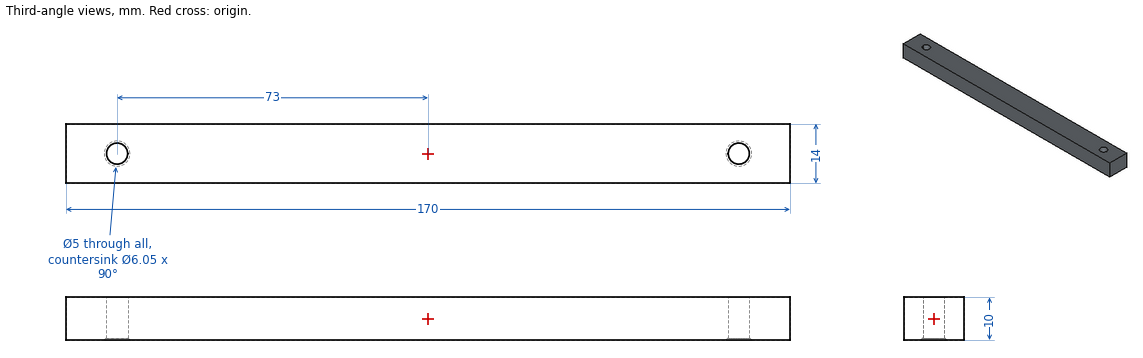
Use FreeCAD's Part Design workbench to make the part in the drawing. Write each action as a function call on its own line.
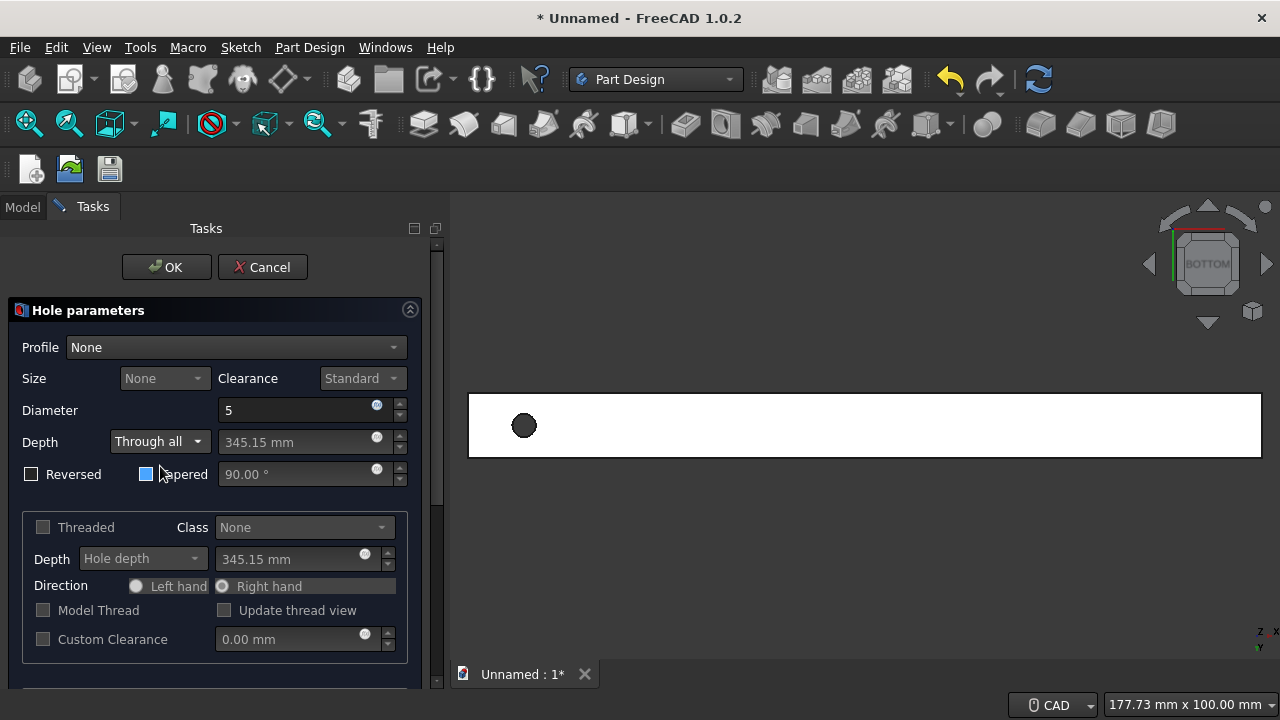
scroll(437, 463, down, 2)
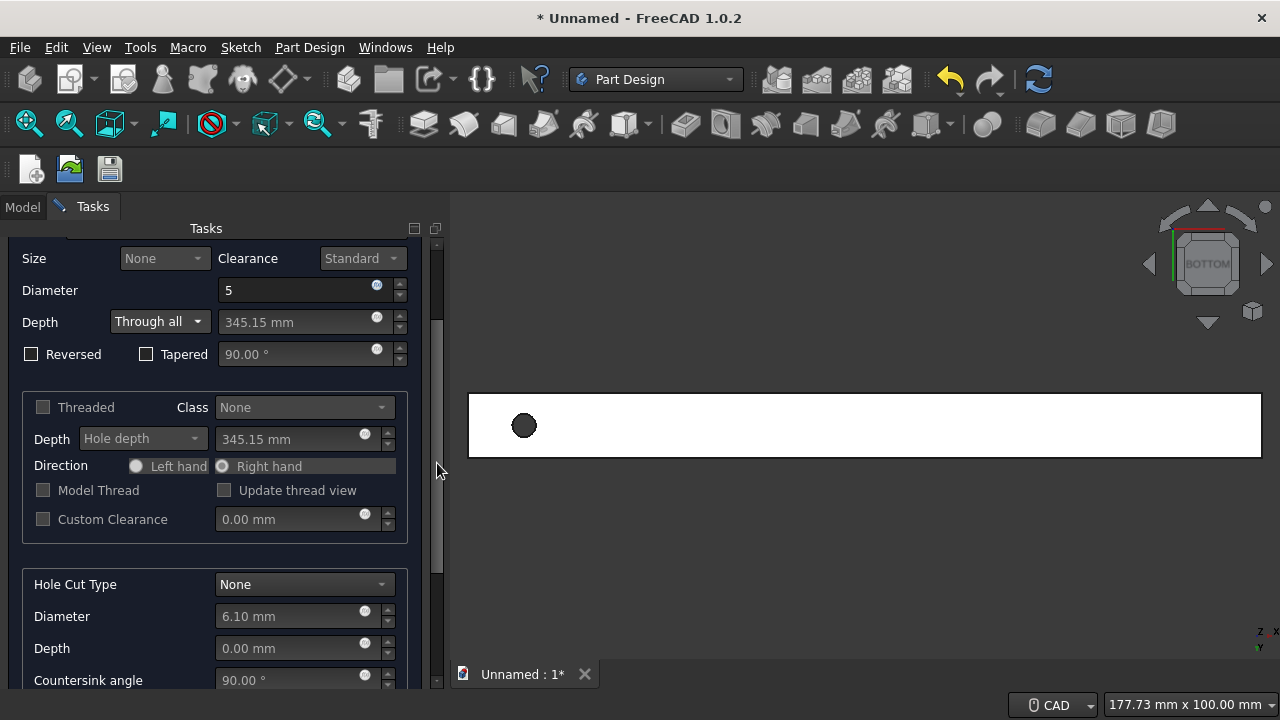
click(306, 584)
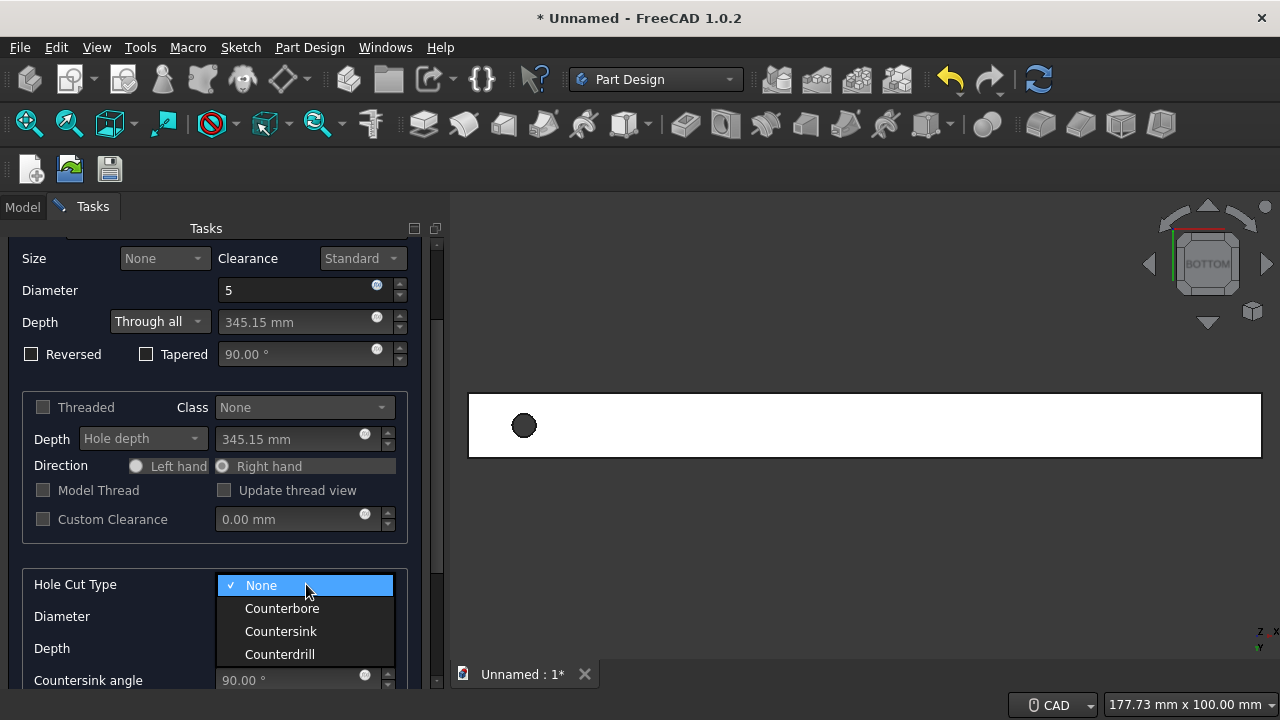
click(304, 632)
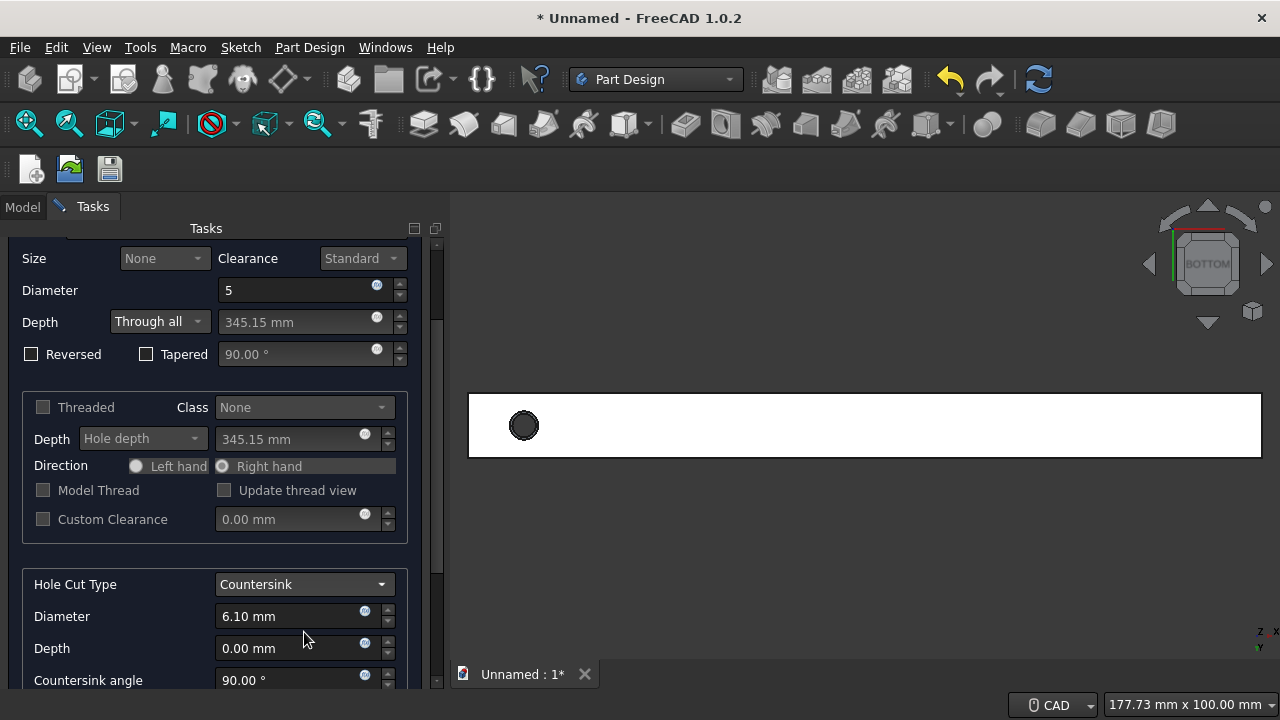
triple_click(298, 616)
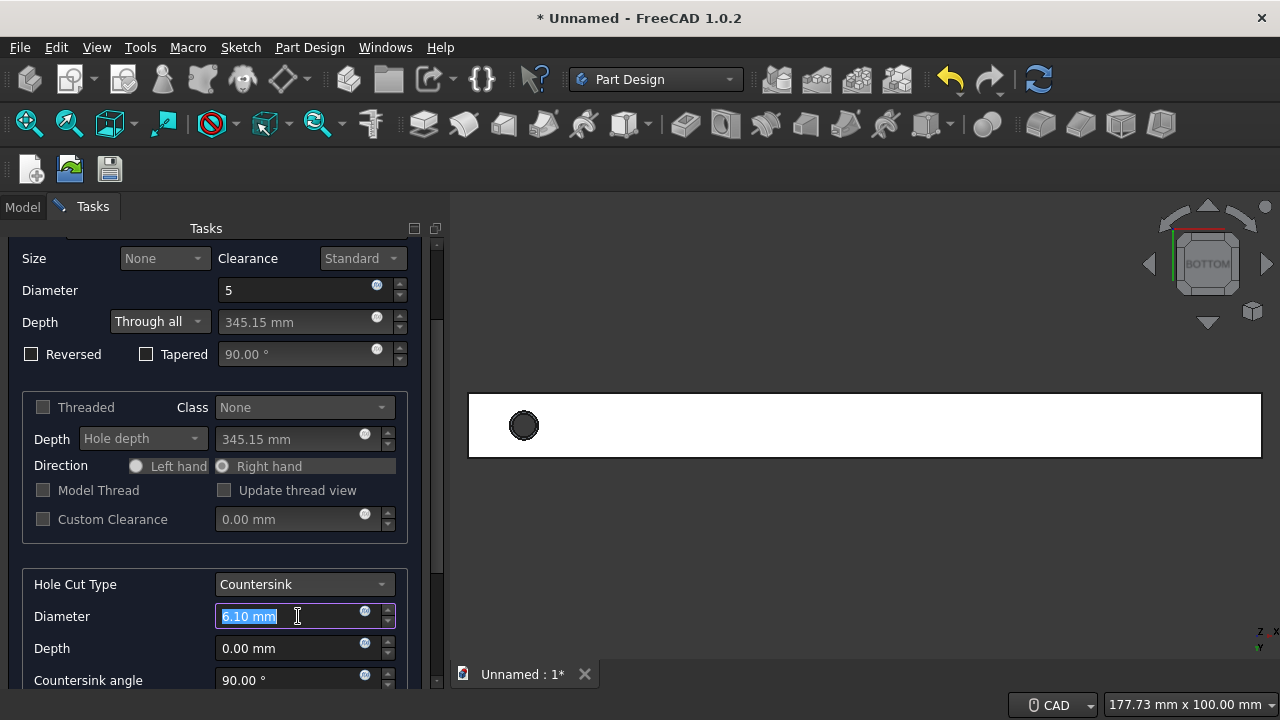
text(6.05)
key(Tab)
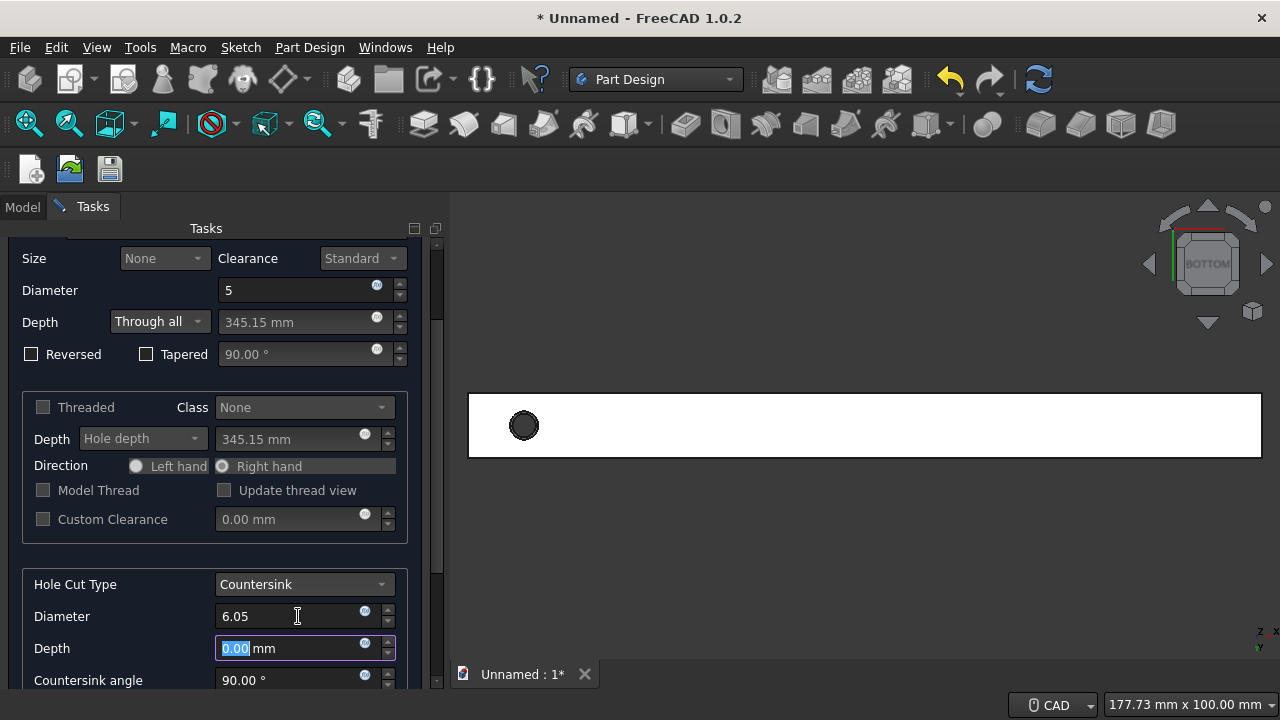
scroll(437, 463, up, 3)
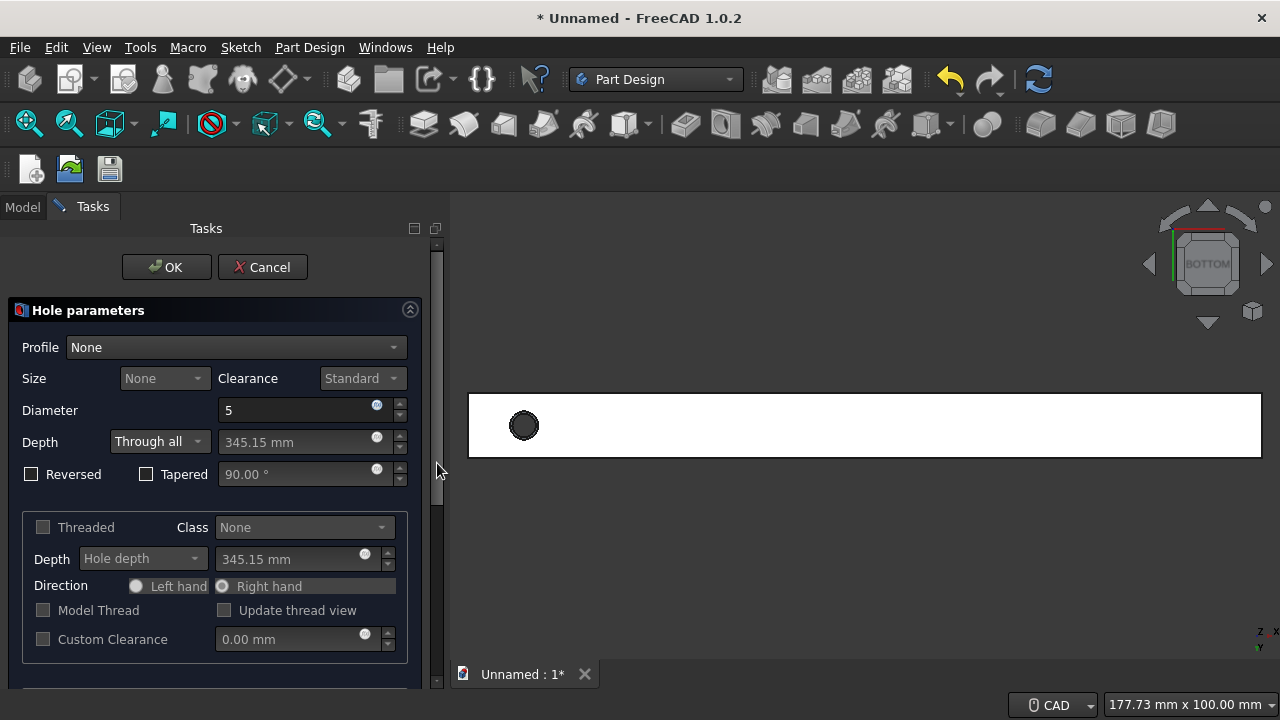
click(167, 267)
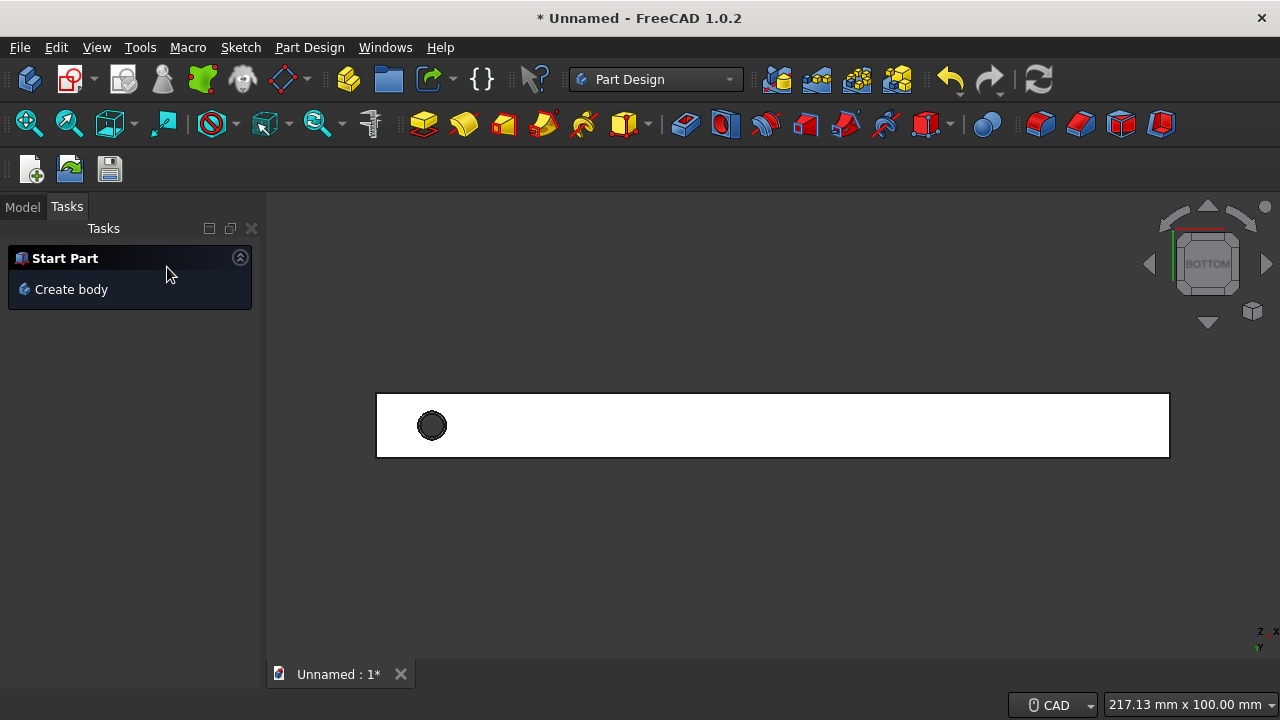
click(23, 206)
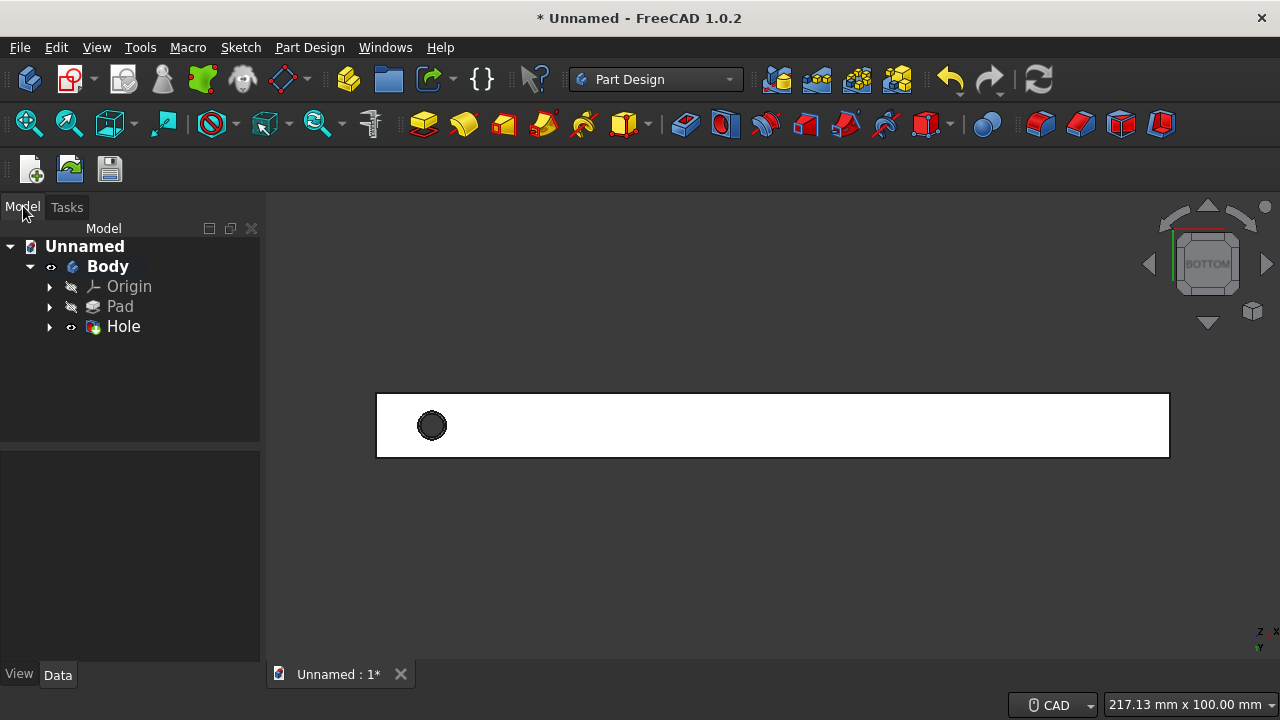
click(116, 327)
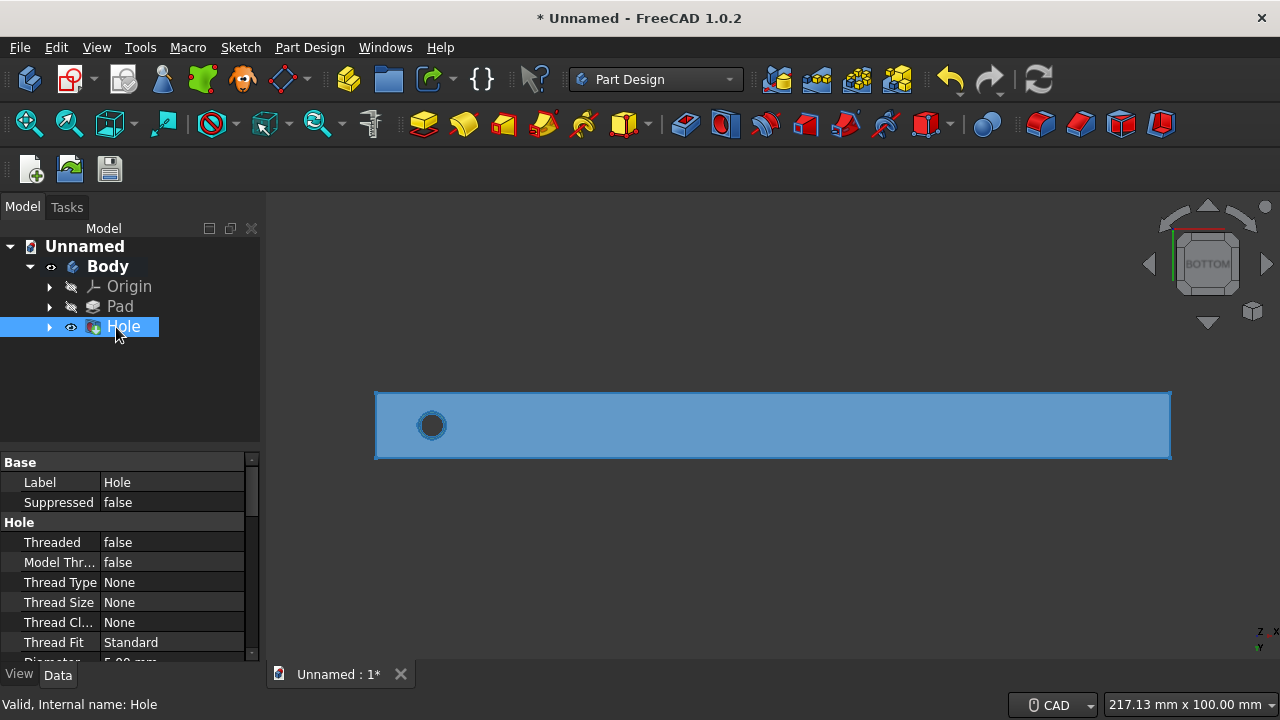
click(778, 80)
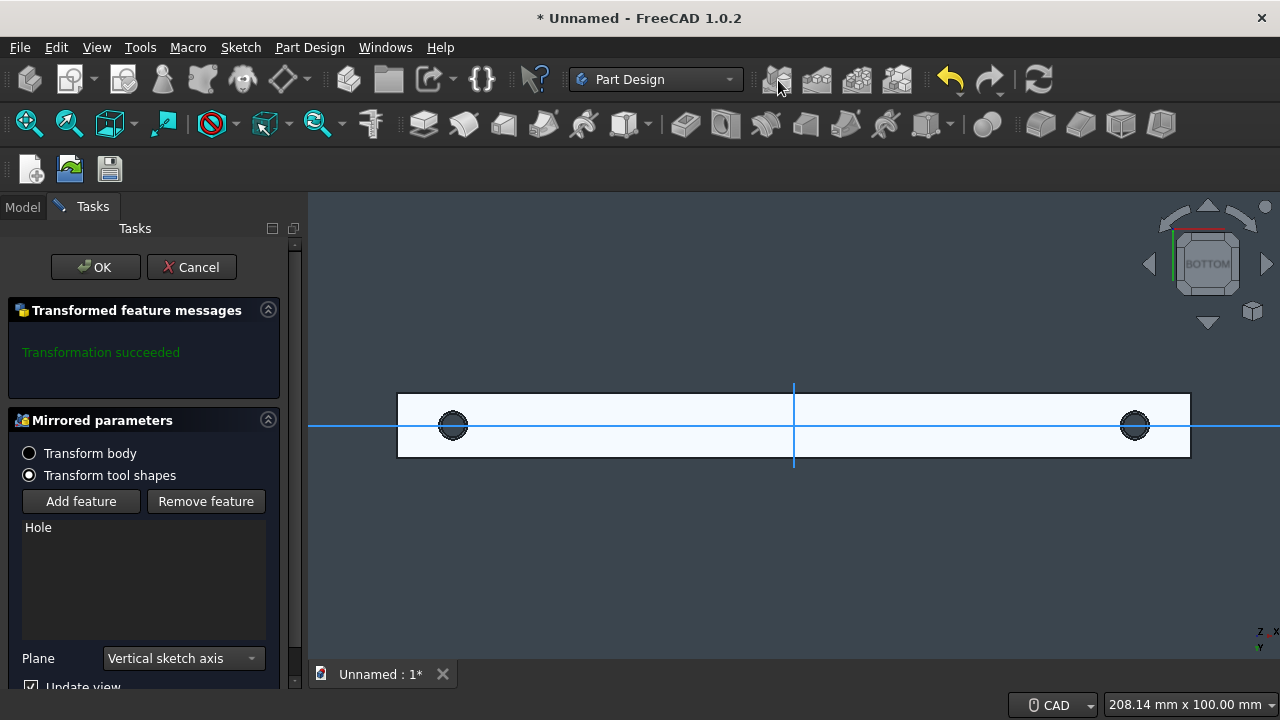
click(184, 658)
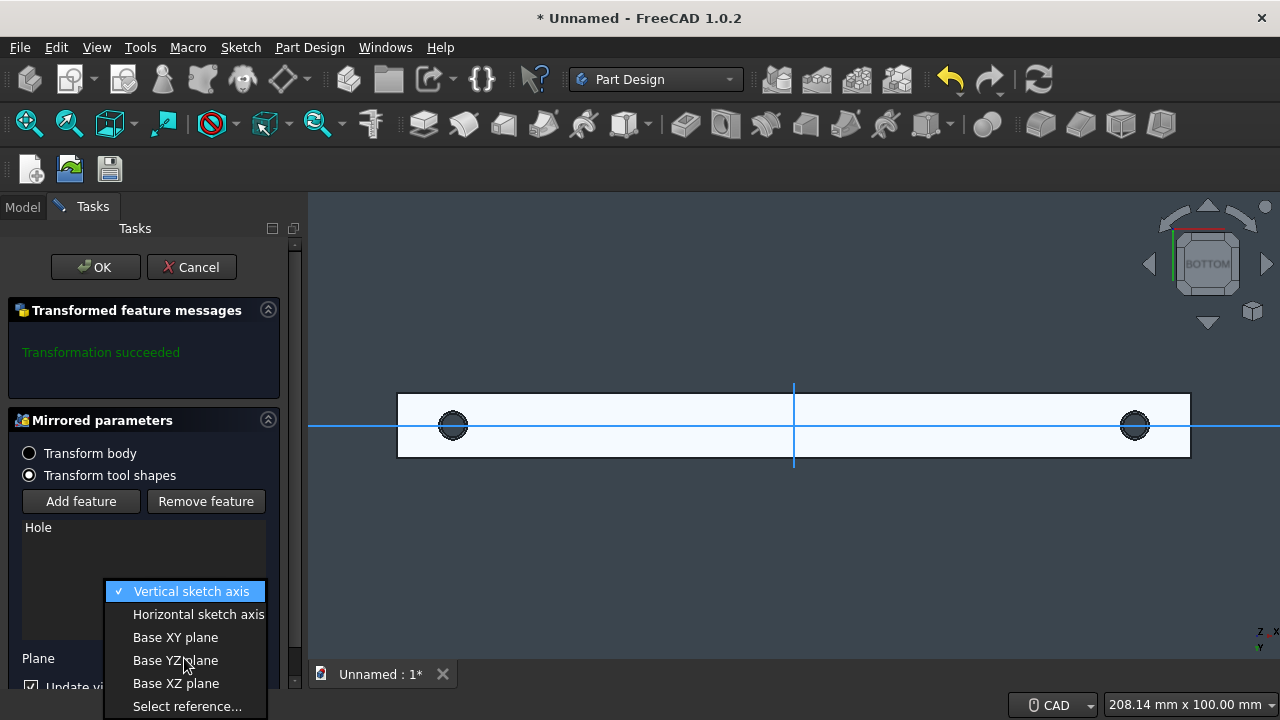
click(184, 660)